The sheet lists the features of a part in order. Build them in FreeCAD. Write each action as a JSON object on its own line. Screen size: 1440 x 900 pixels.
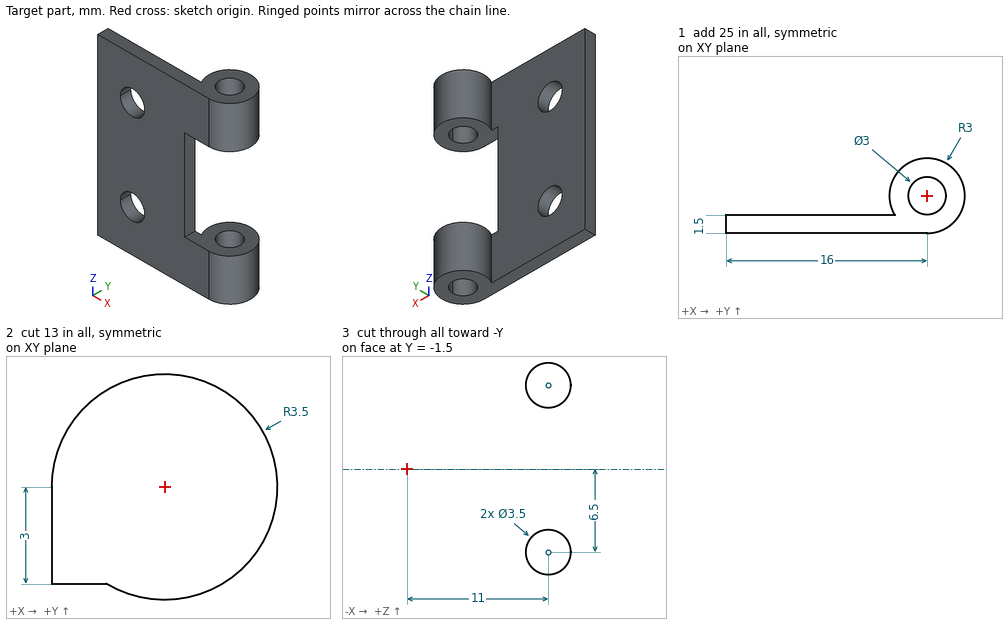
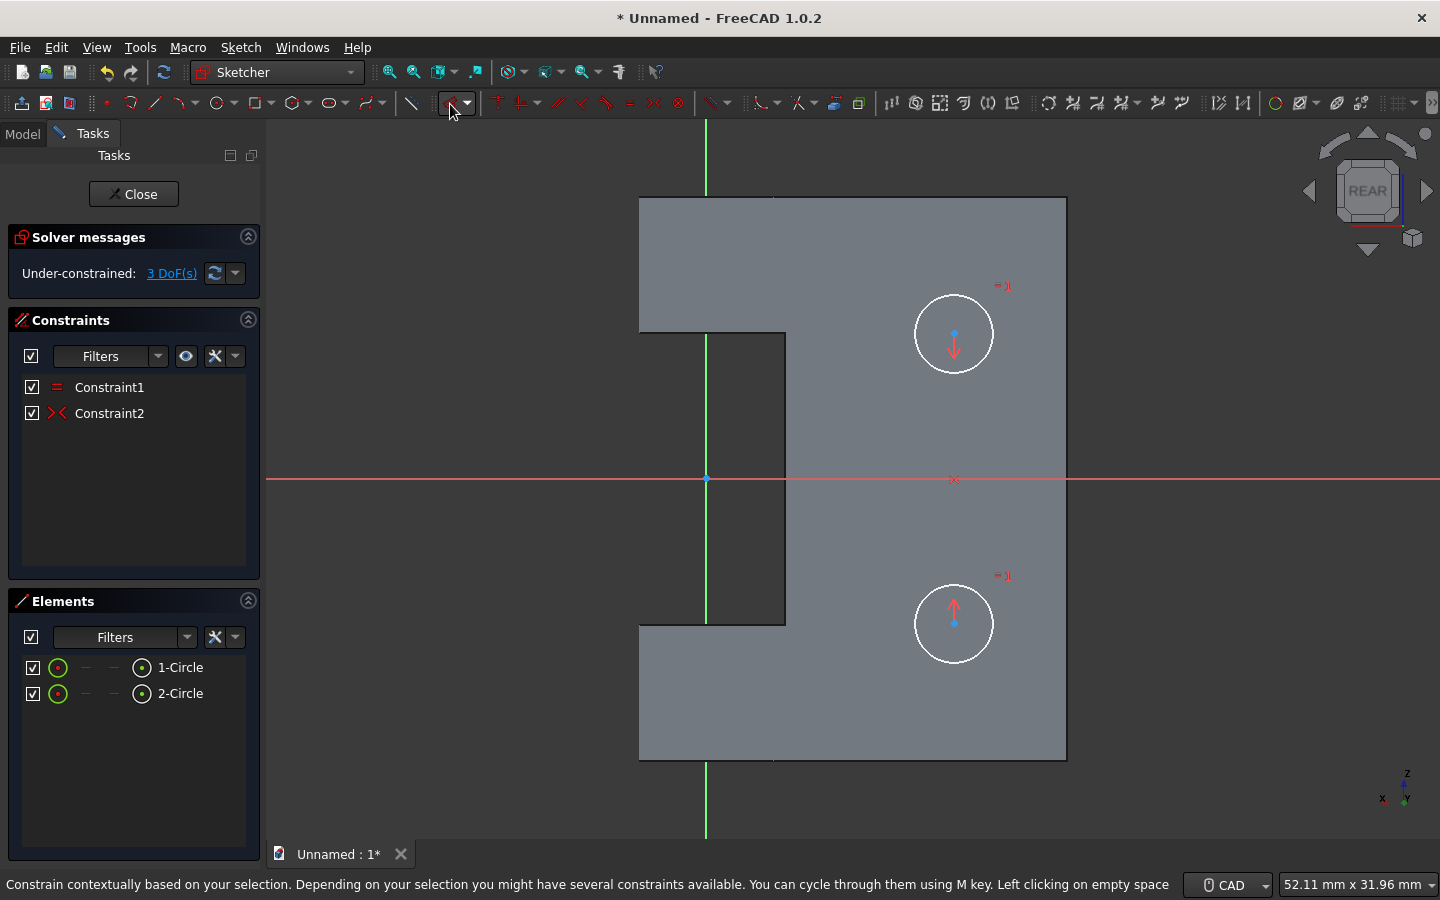
{"action": "left_click", "coordinate": [981, 596]}
{"action": "left_click", "coordinate": [1003, 573]}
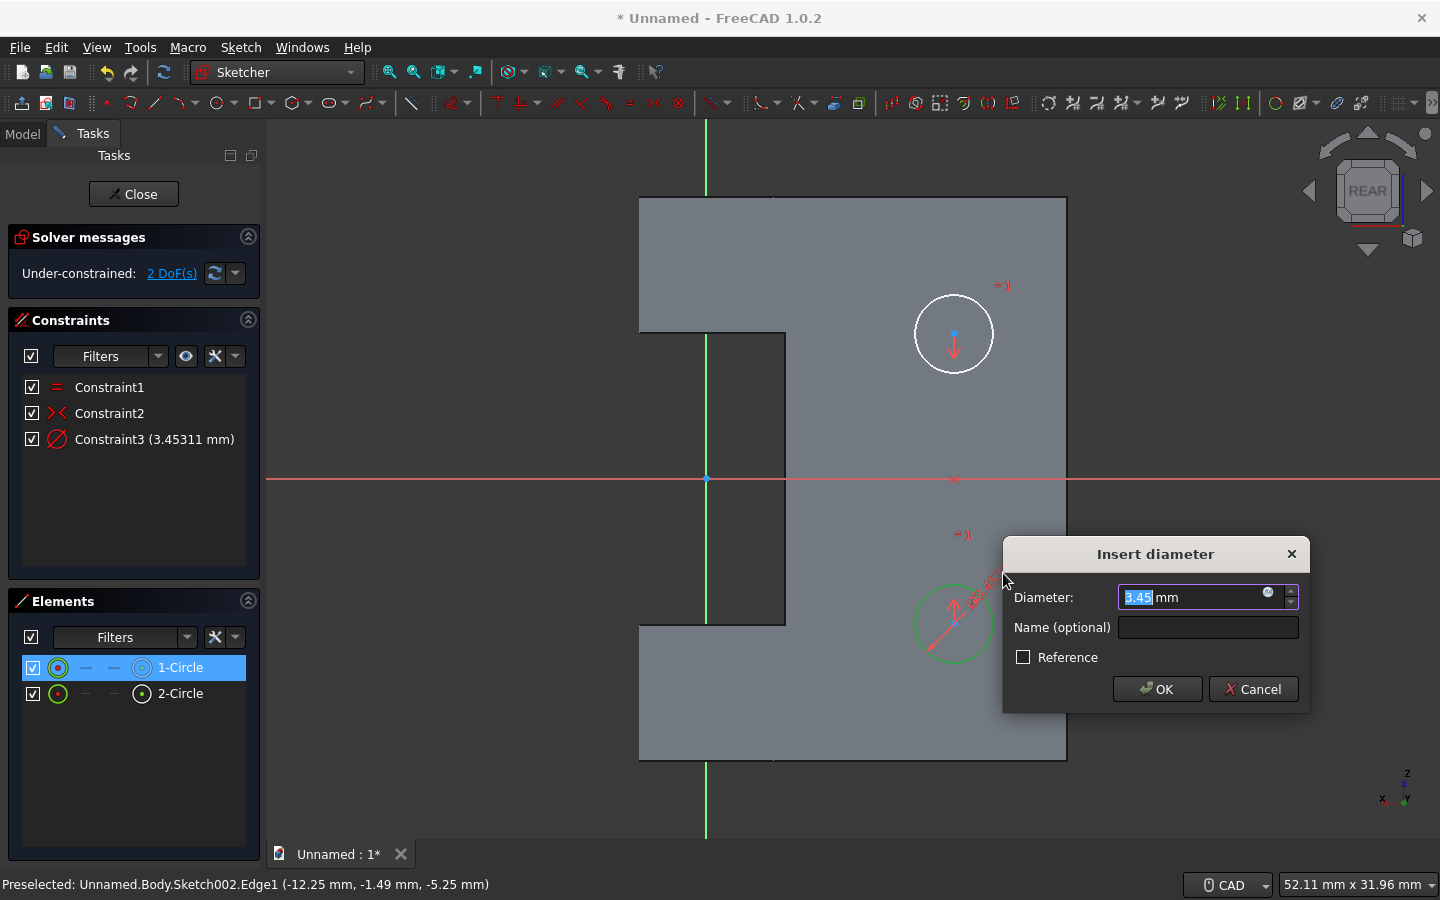
{"action": "type", "text": "3.5"}
{"action": "key", "text": "Return"}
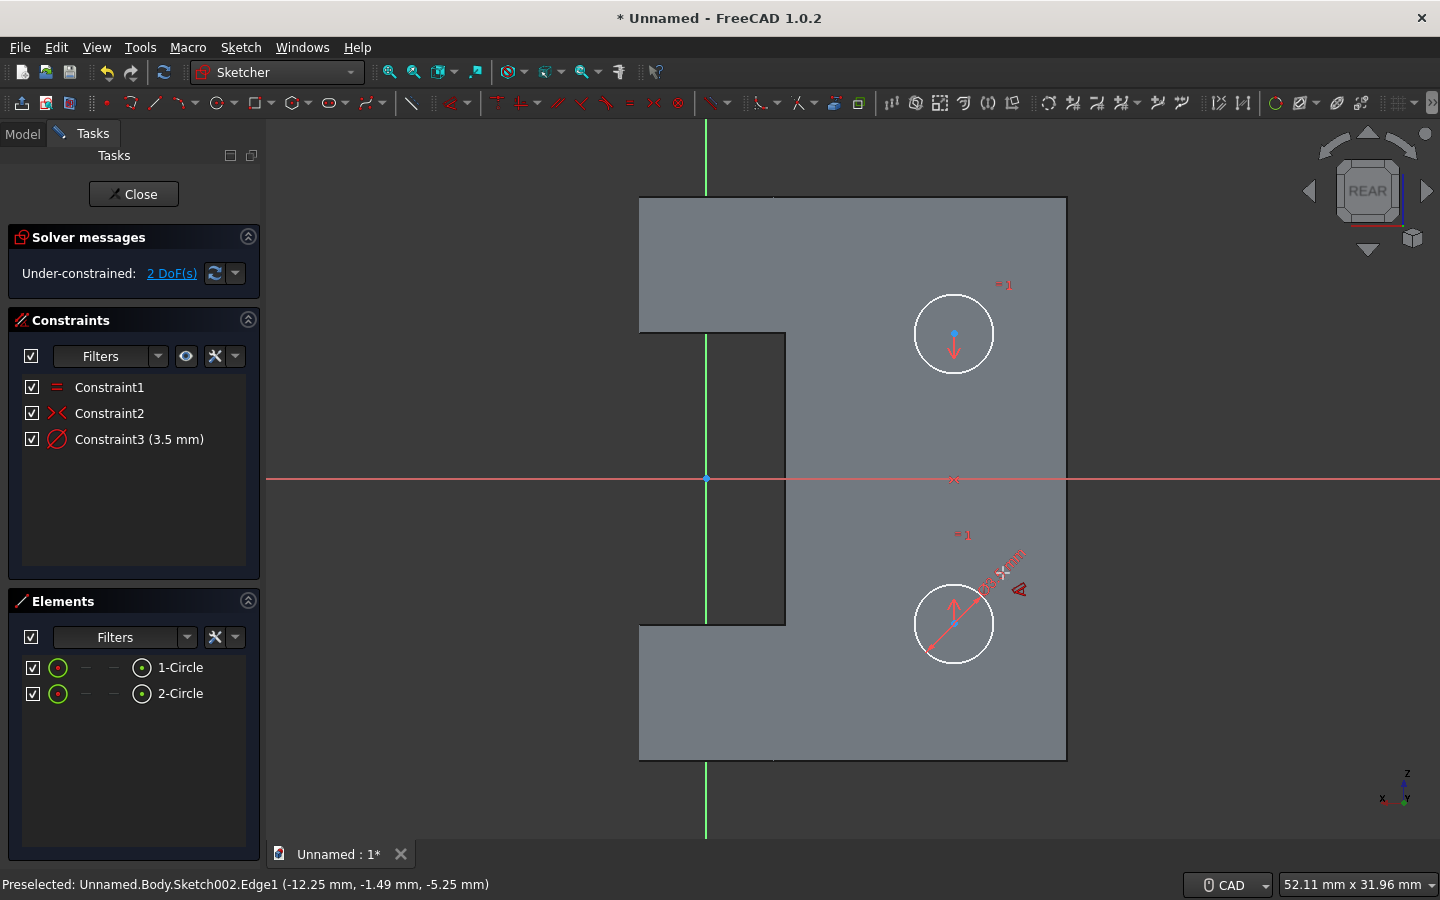
{"action": "left_click", "coordinate": [954, 624]}
{"action": "left_click", "coordinate": [830, 658]}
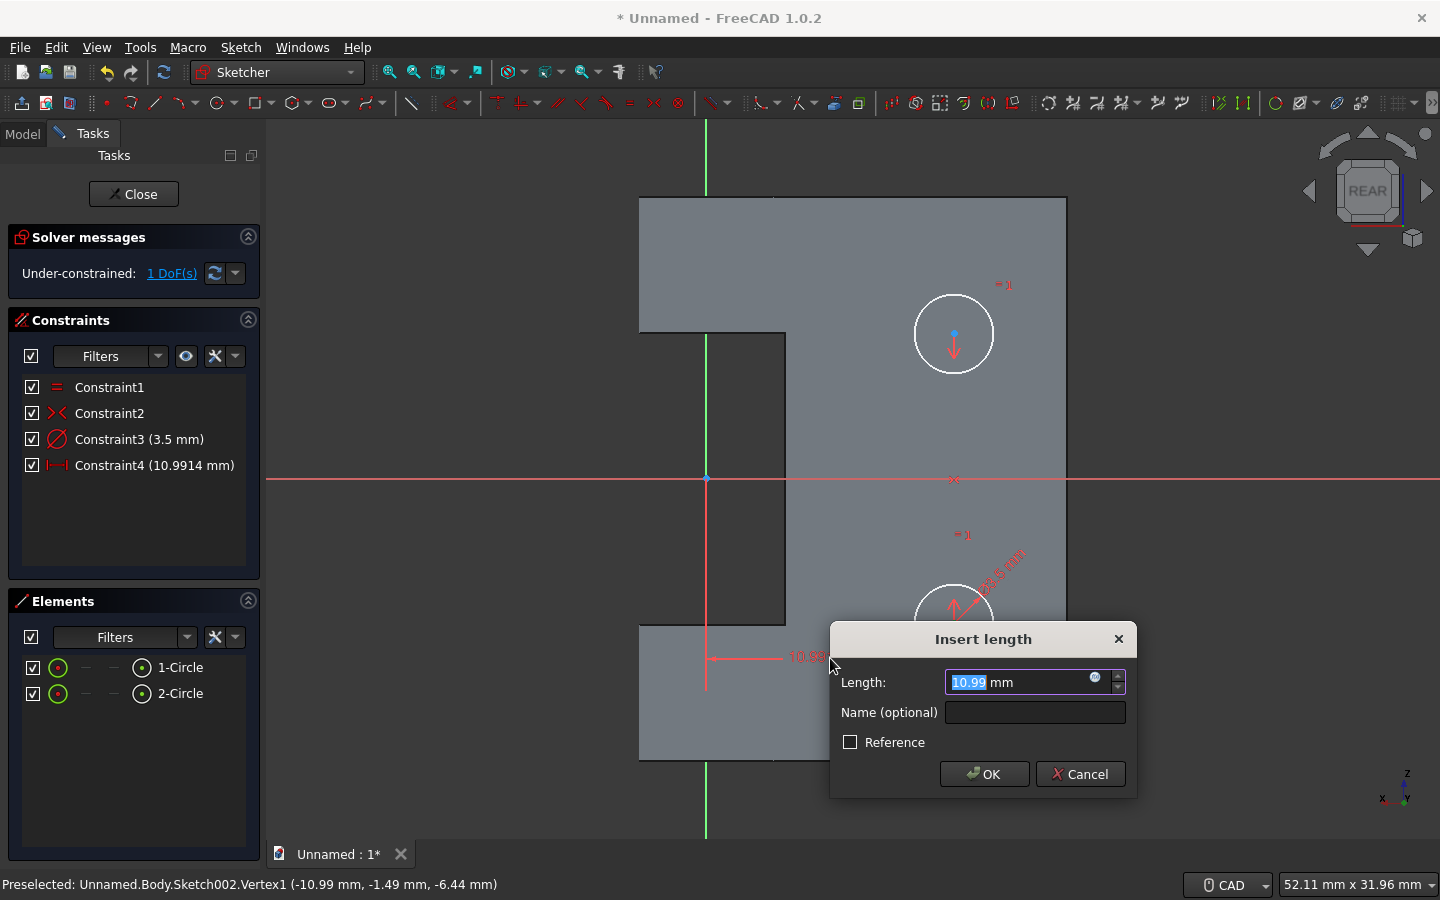
{"action": "type", "text": "11"}
{"action": "key", "text": "Return"}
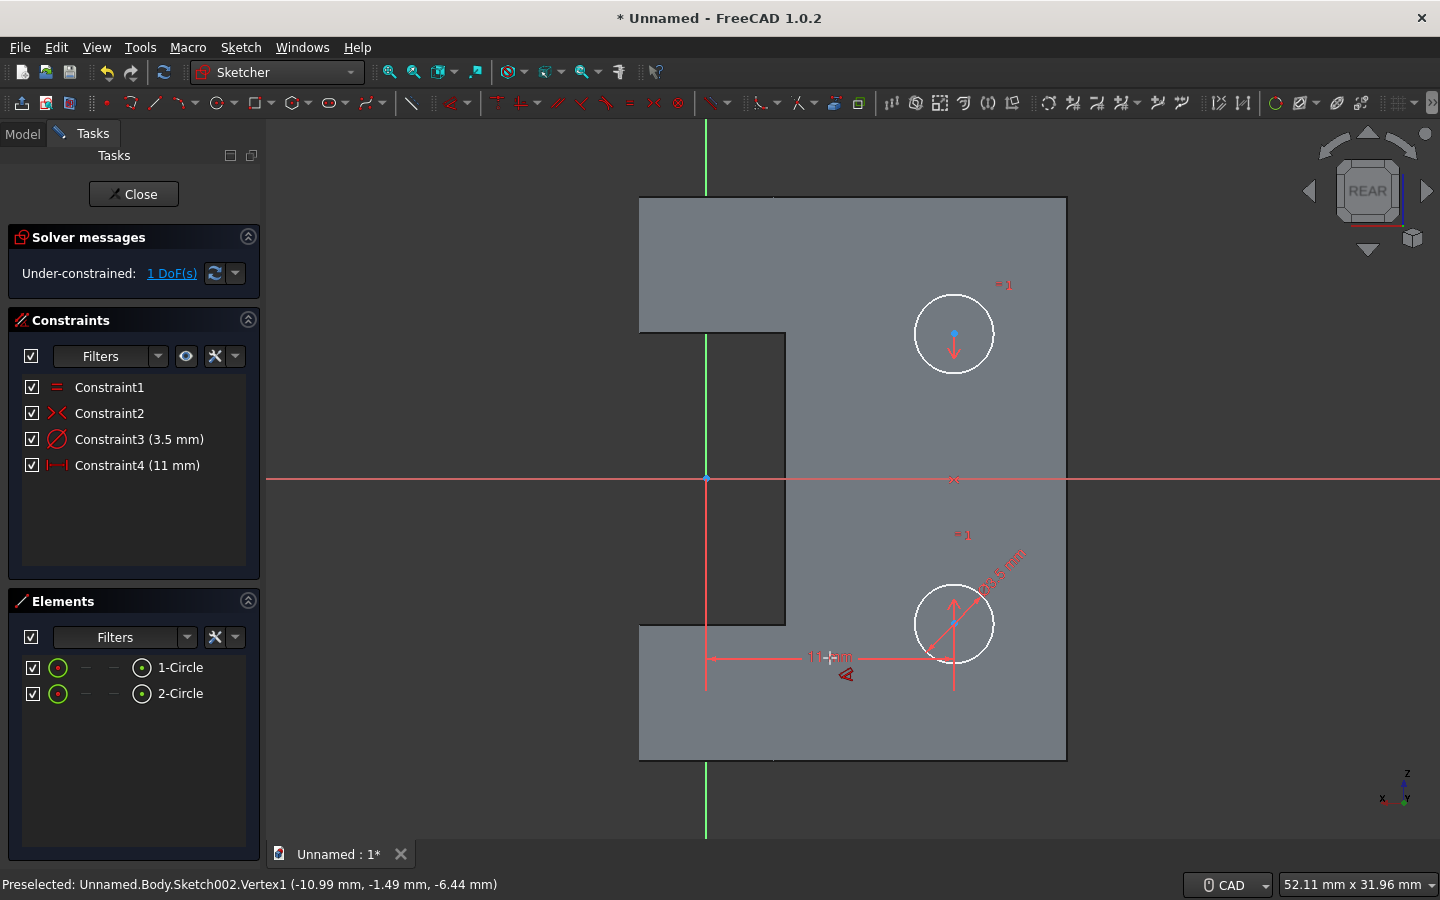
{"action": "left_click", "coordinate": [954, 624]}
{"action": "left_click", "coordinate": [672, 552]}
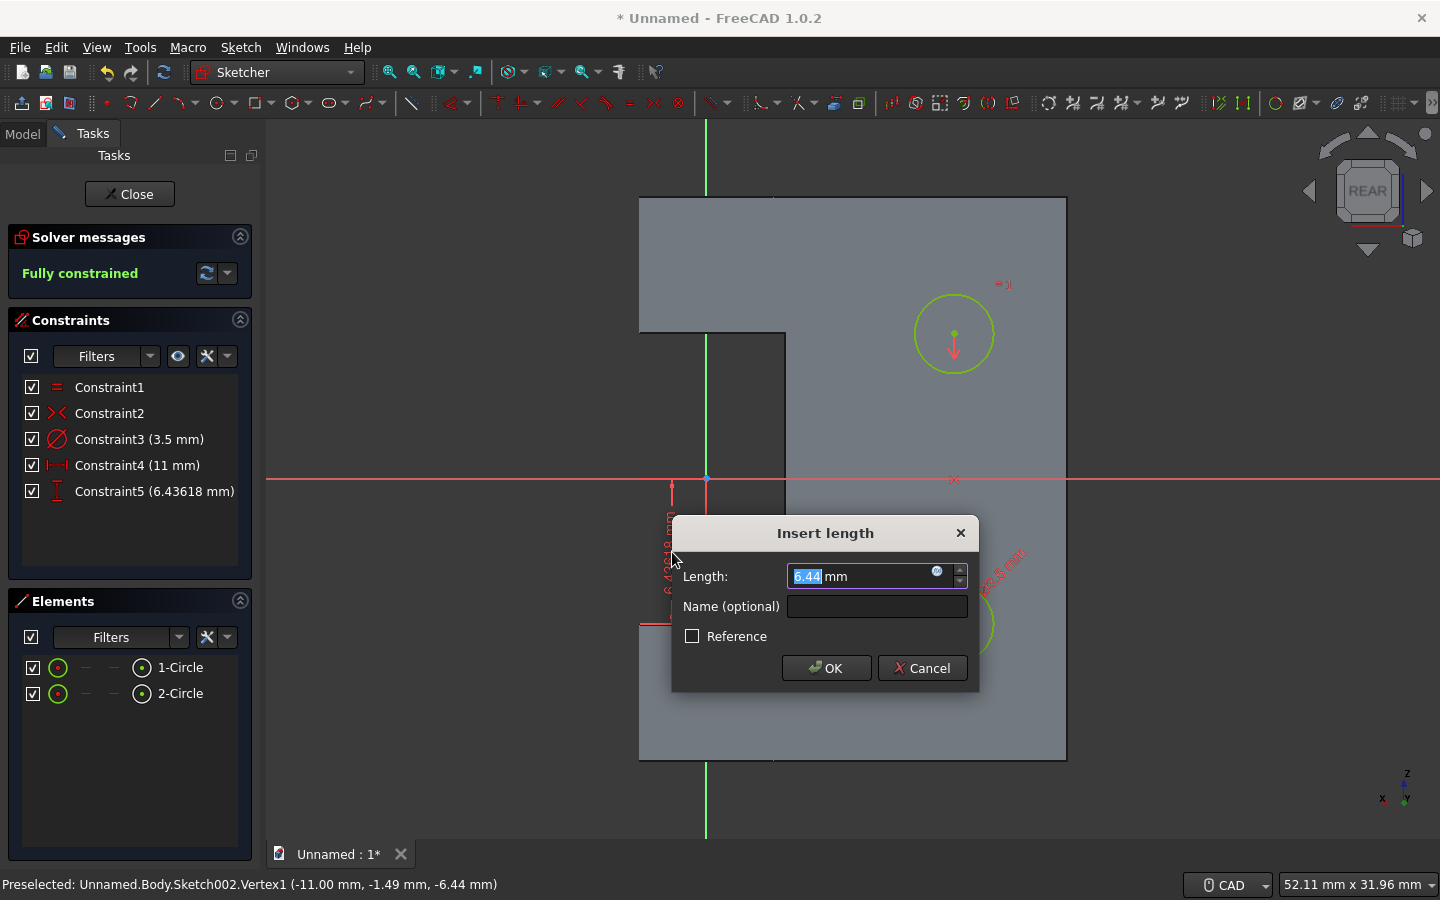
{"action": "type", "text": "6.5"}
{"action": "key", "text": "Return"}
{"action": "key", "text": "Escape"}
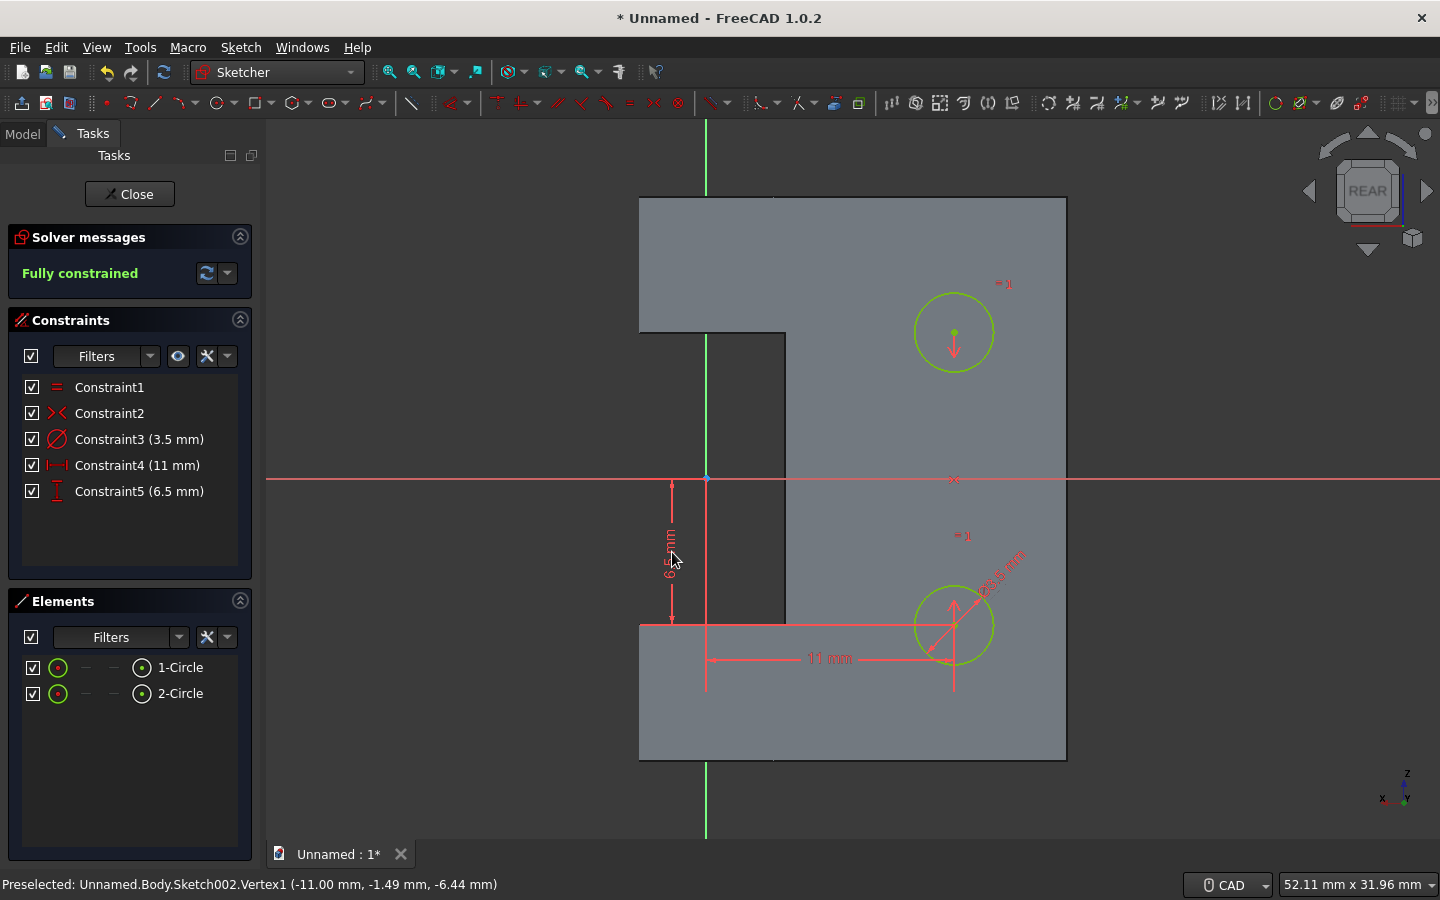
{"action": "left_click", "coordinate": [130, 194]}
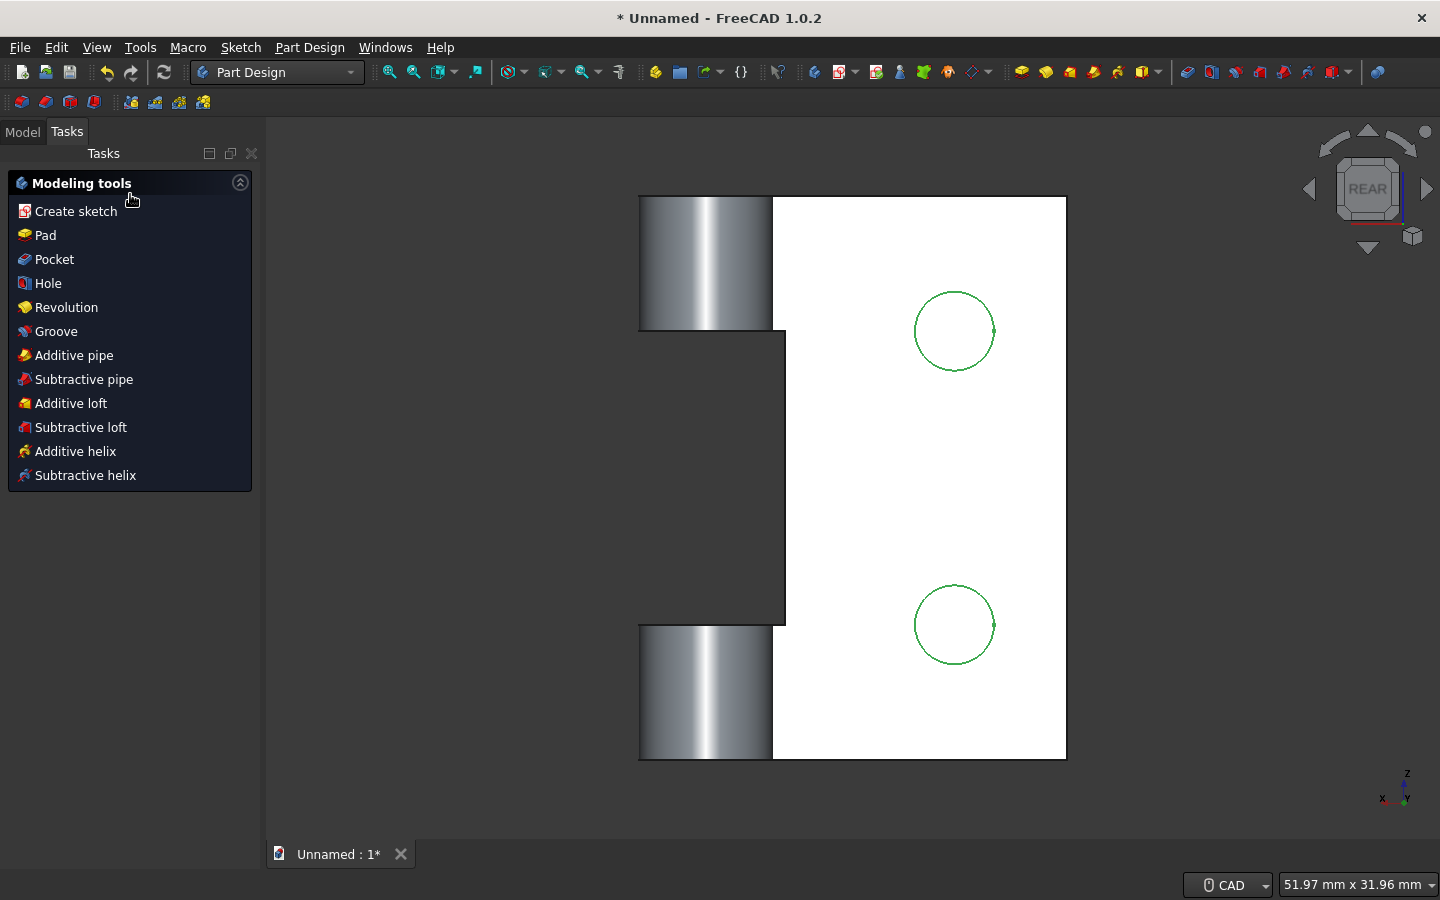
{"action": "left_click", "coordinate": [1188, 72]}